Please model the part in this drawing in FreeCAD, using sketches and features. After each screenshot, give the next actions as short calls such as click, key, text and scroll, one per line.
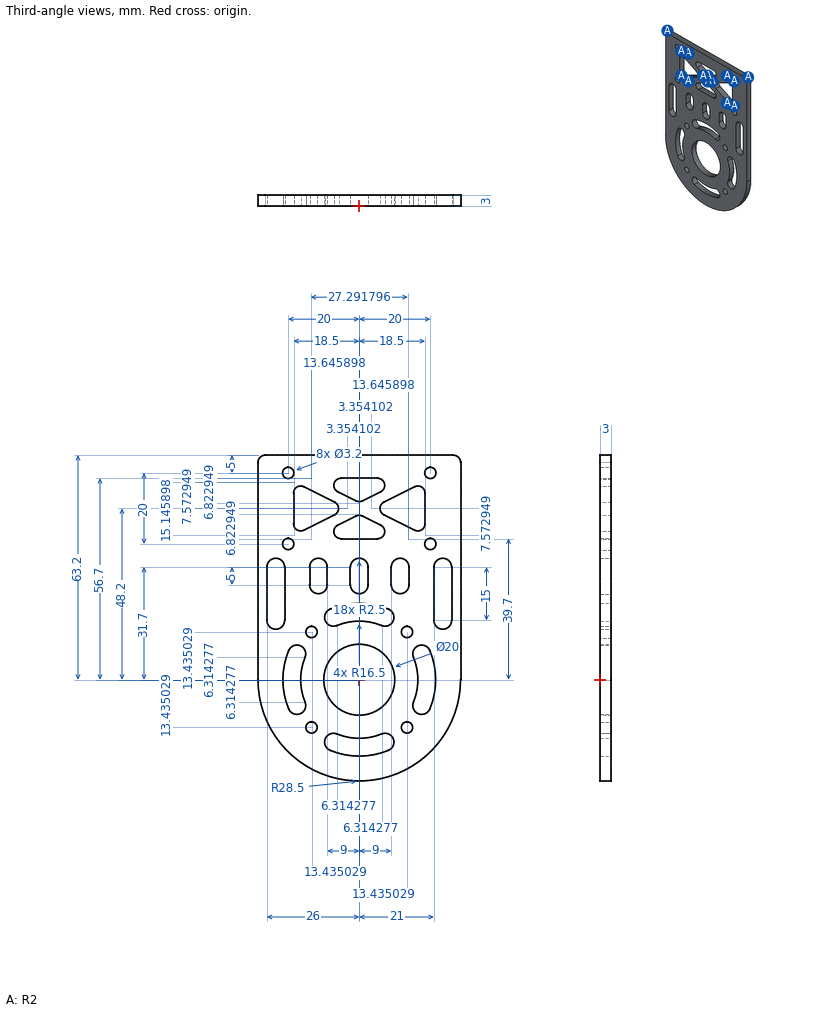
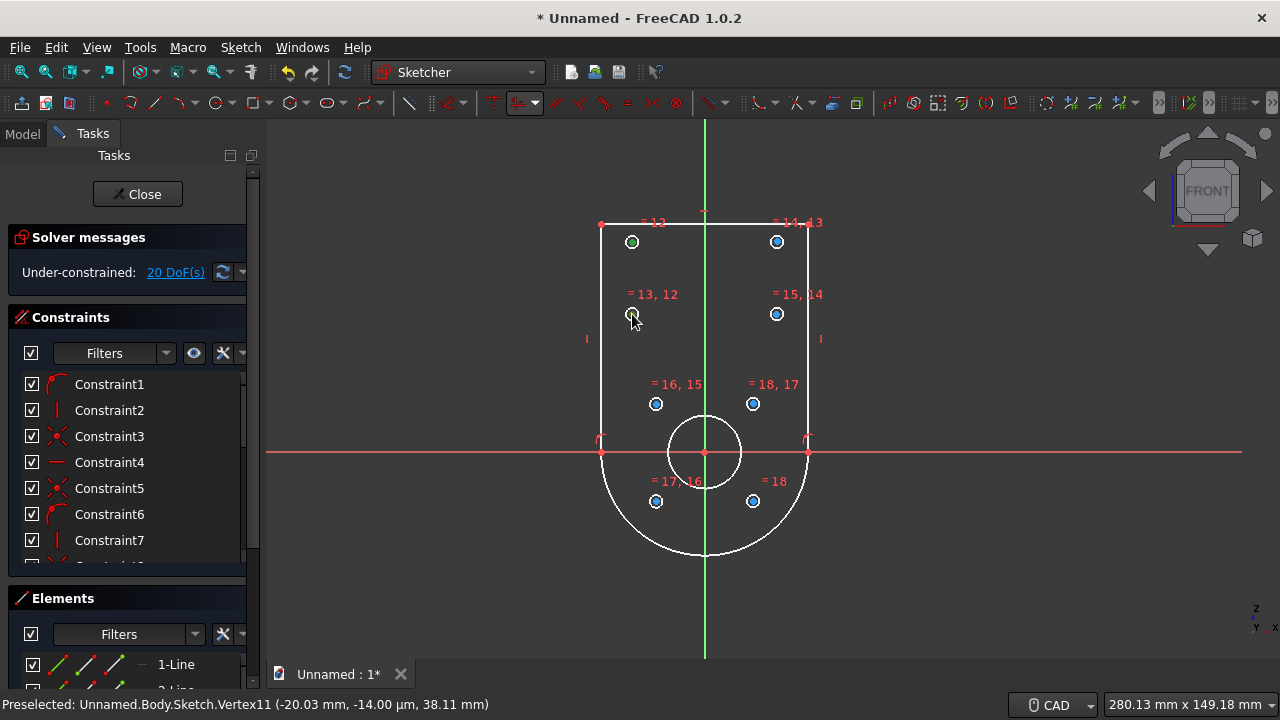
click(538, 104)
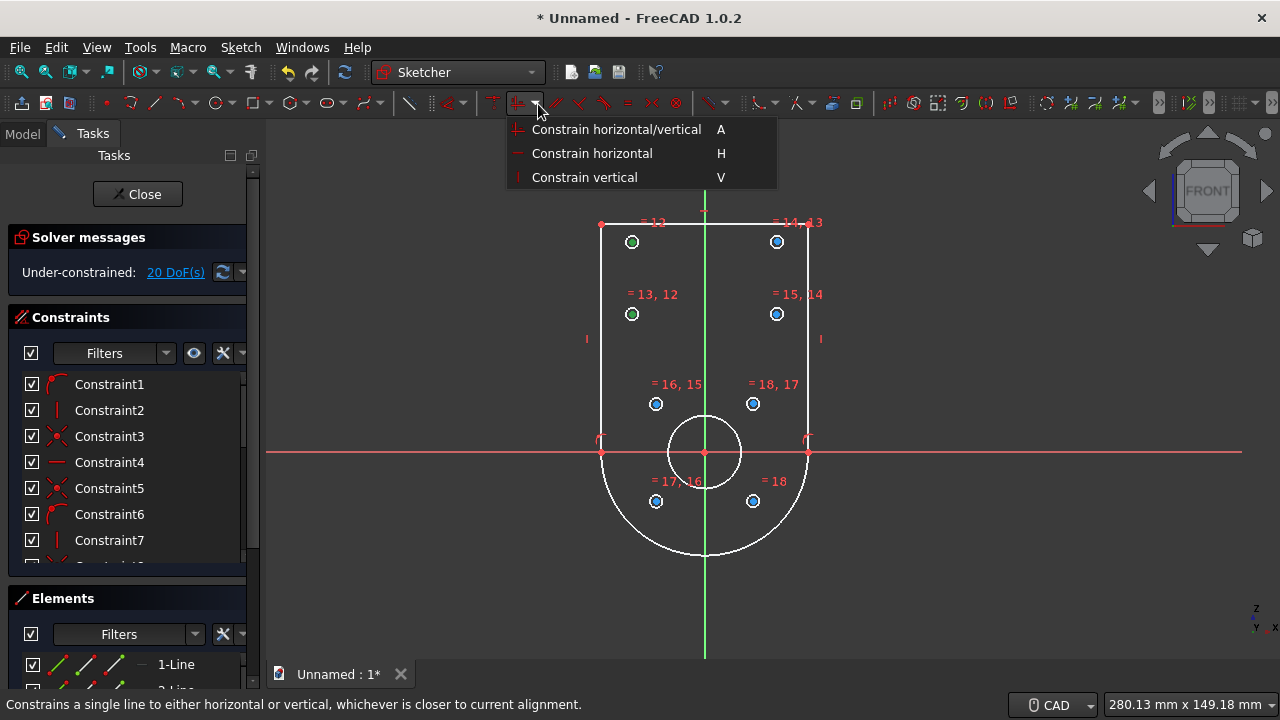
click(642, 177)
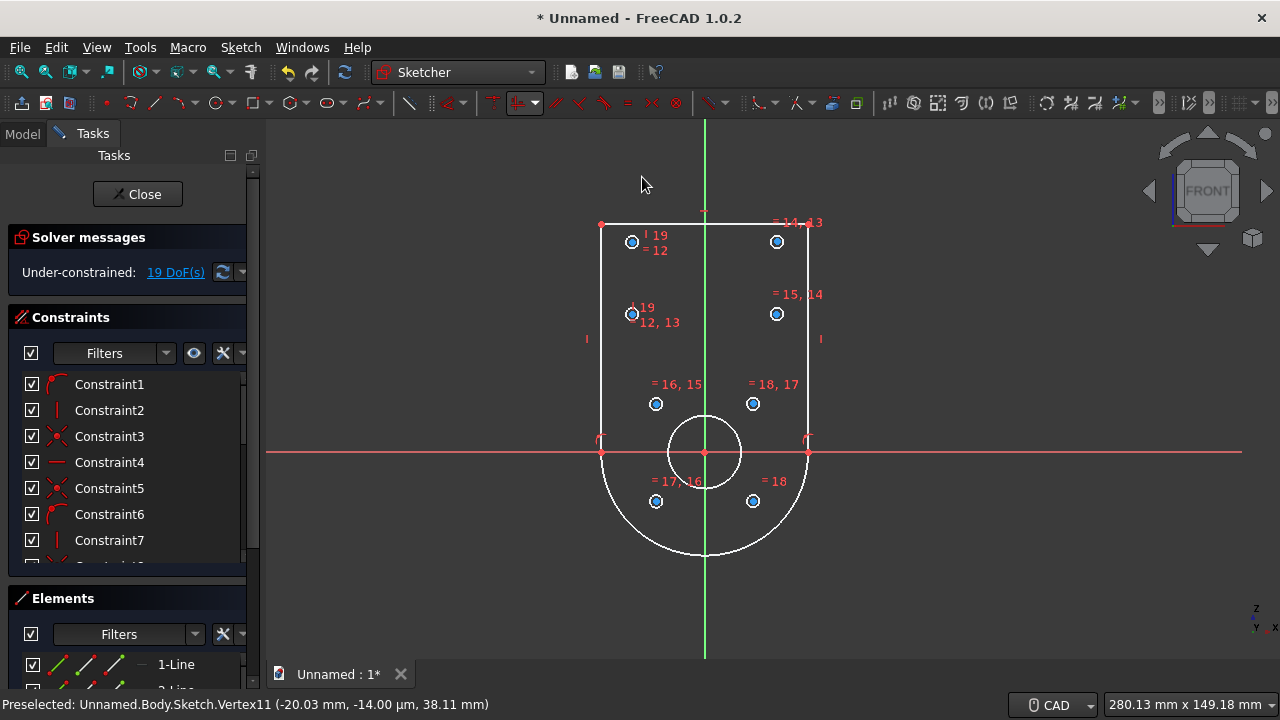
click(632, 242)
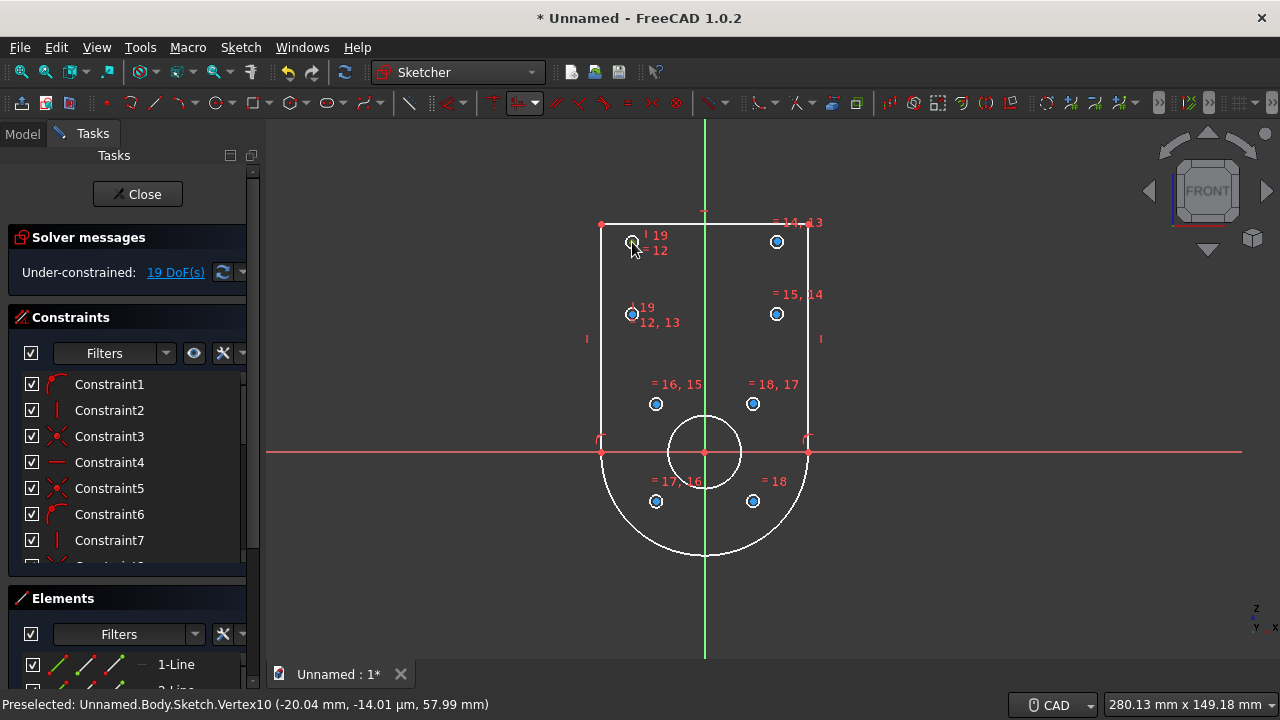
click(777, 242)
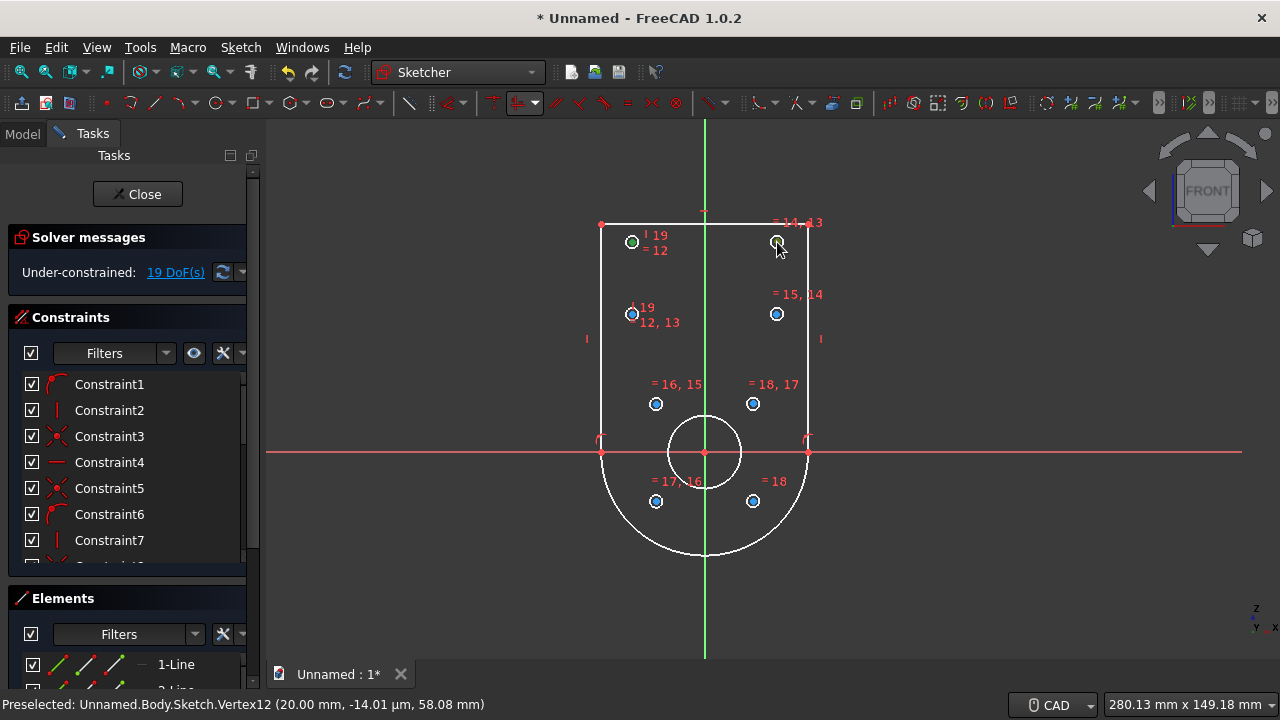
click(538, 104)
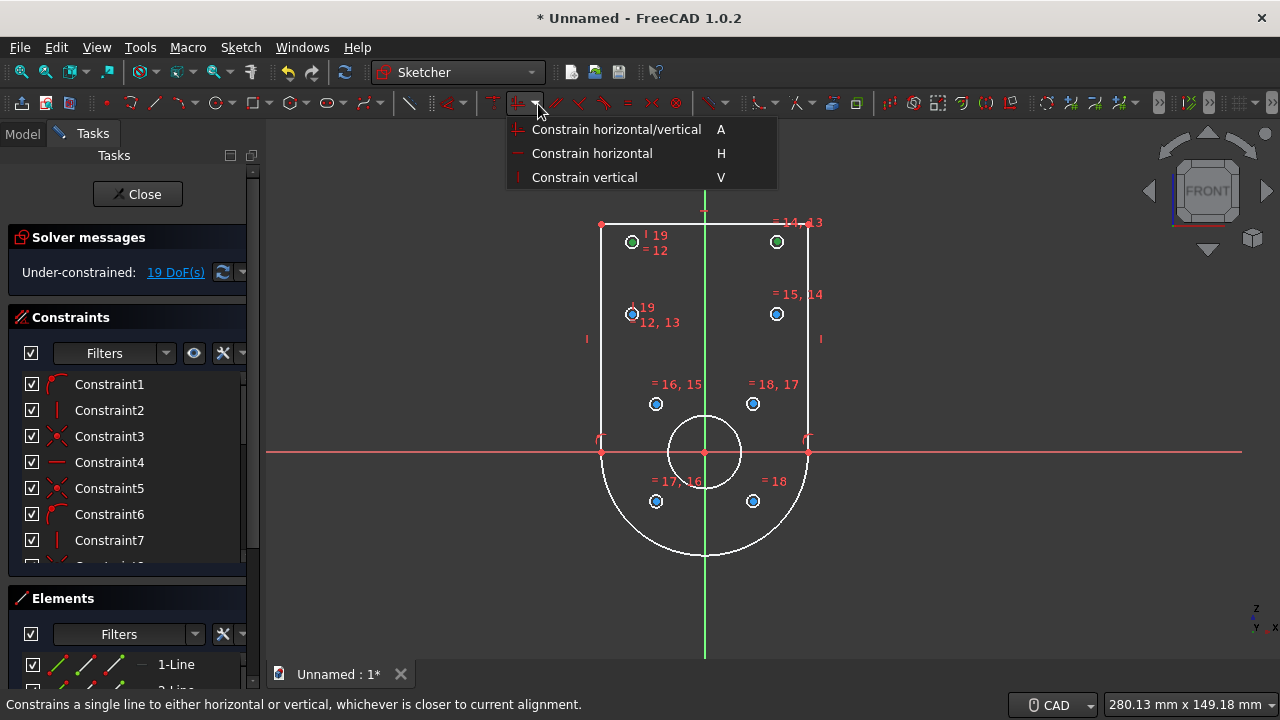
click(642, 153)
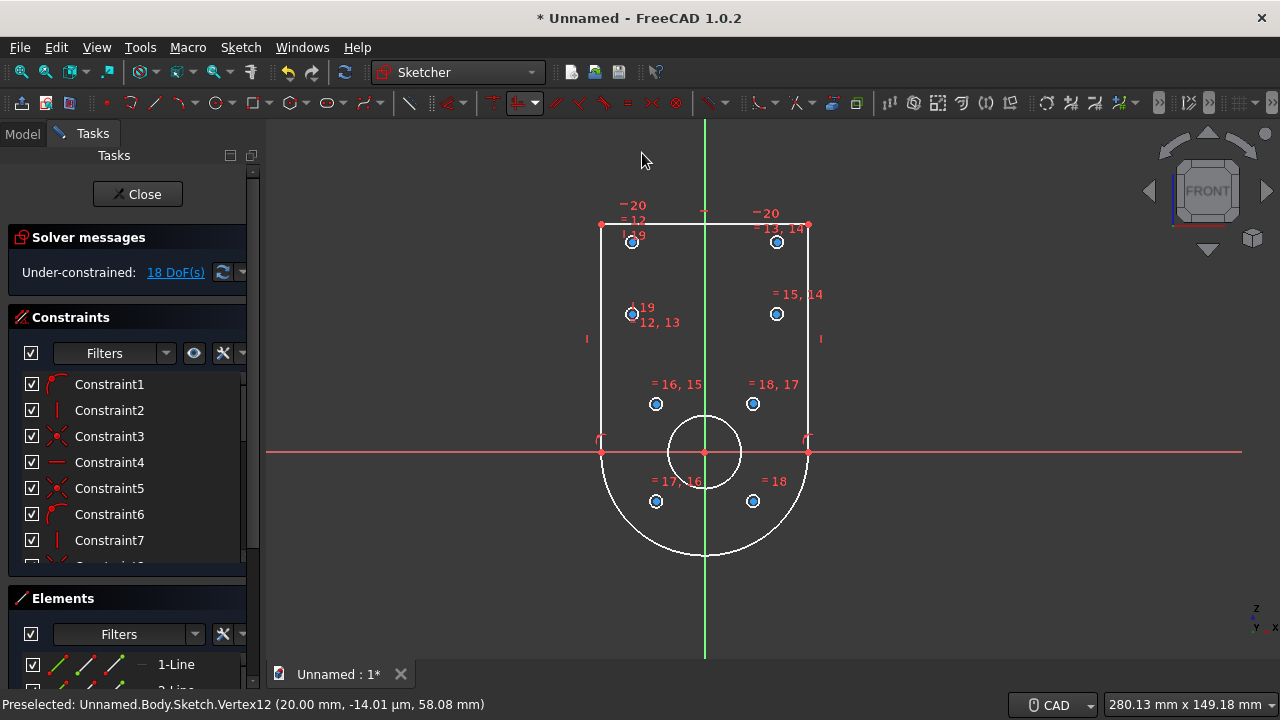
click(777, 242)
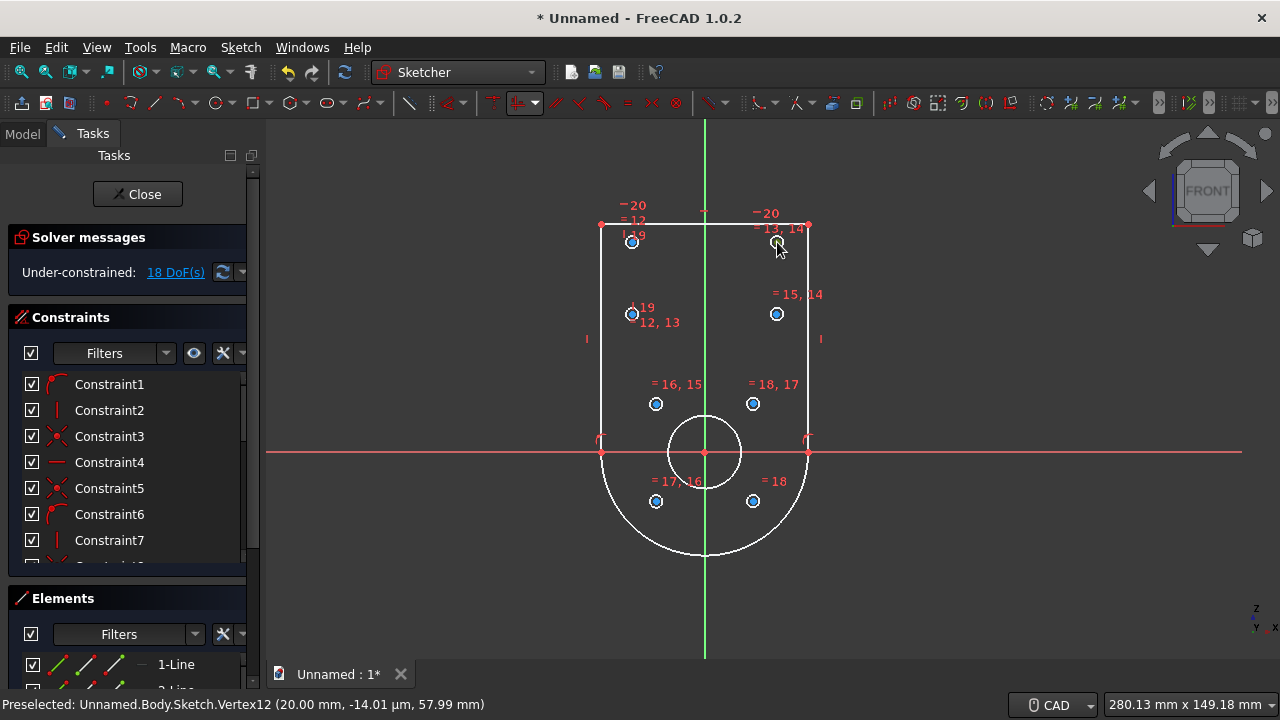
click(777, 314)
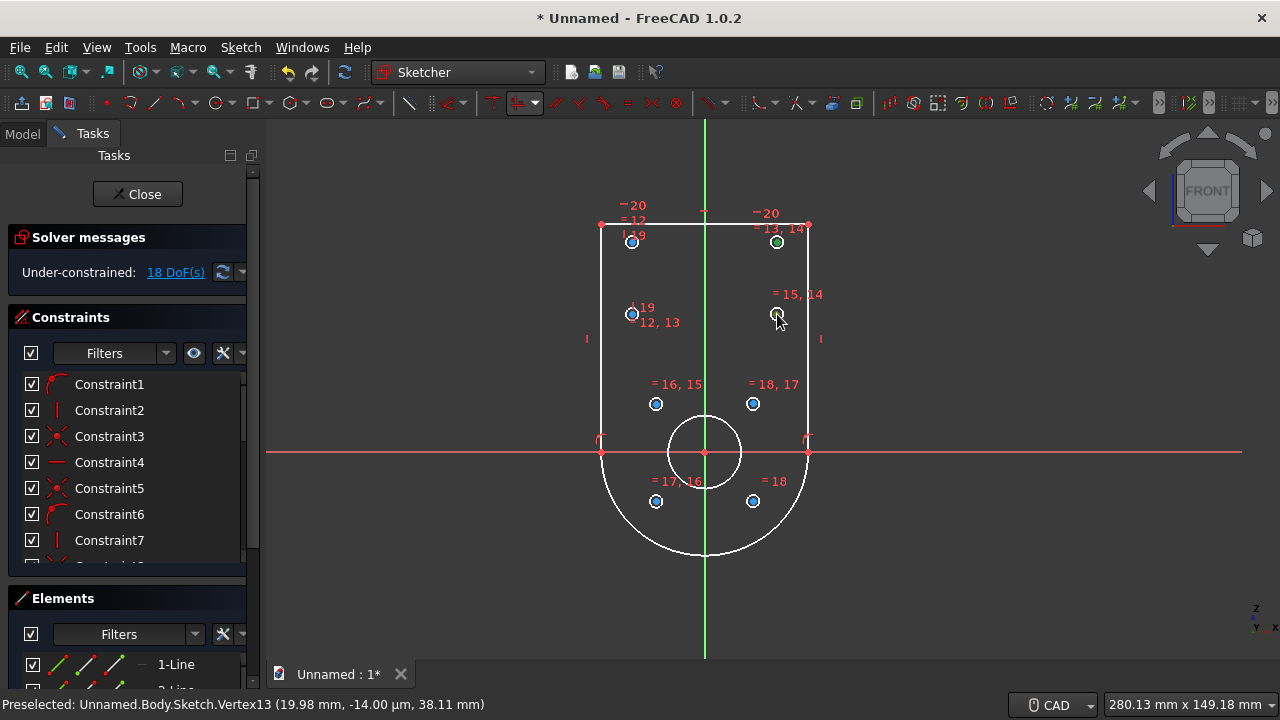
key(v)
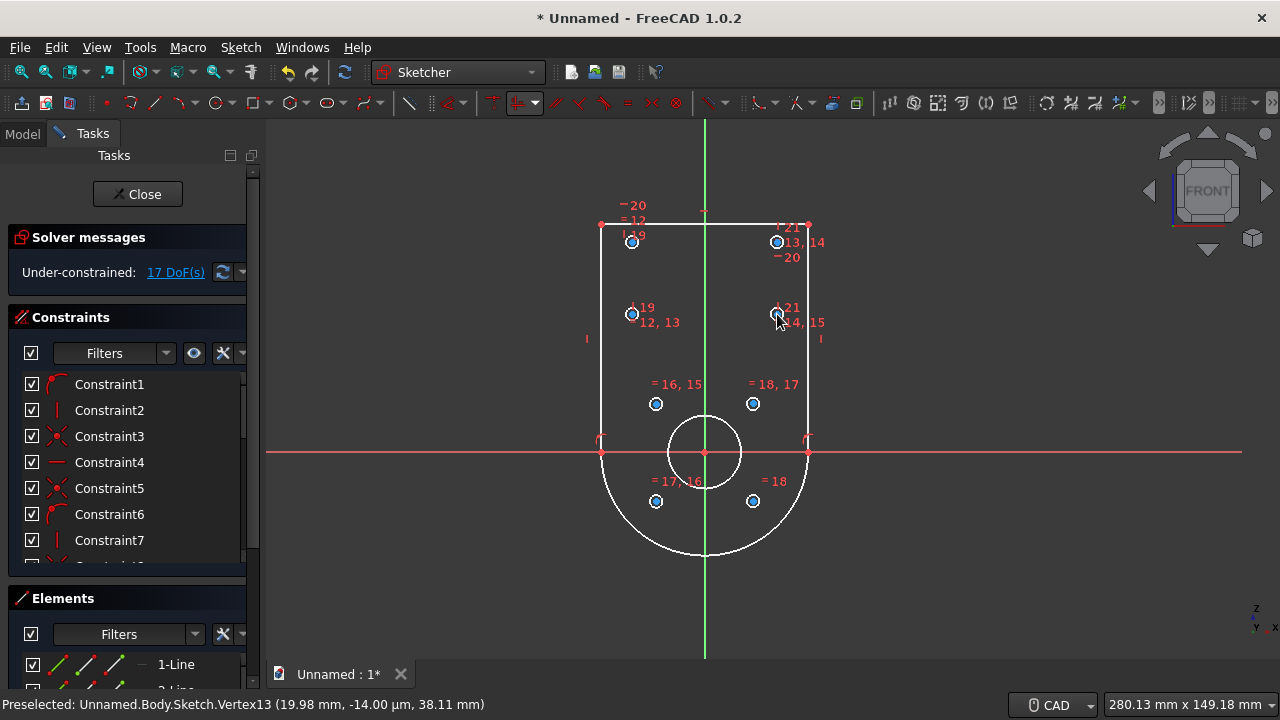
scroll(632, 314, up, 4)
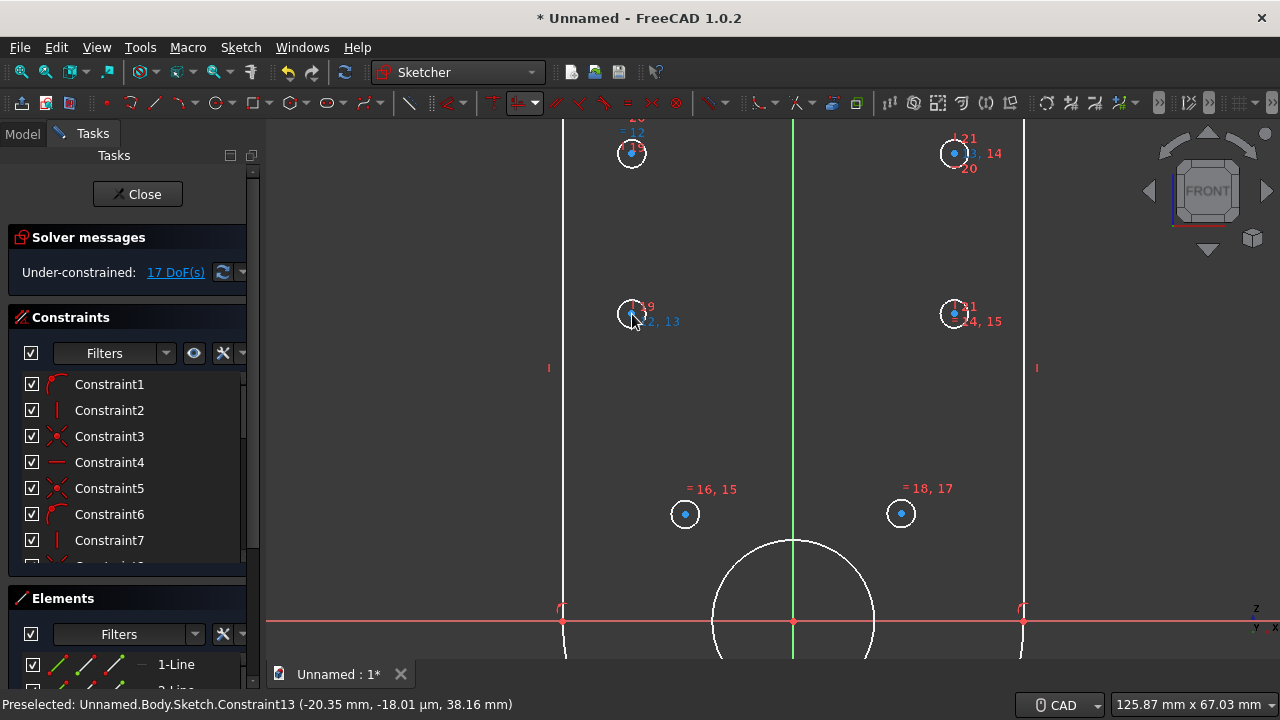
scroll(632, 314, up, 4)